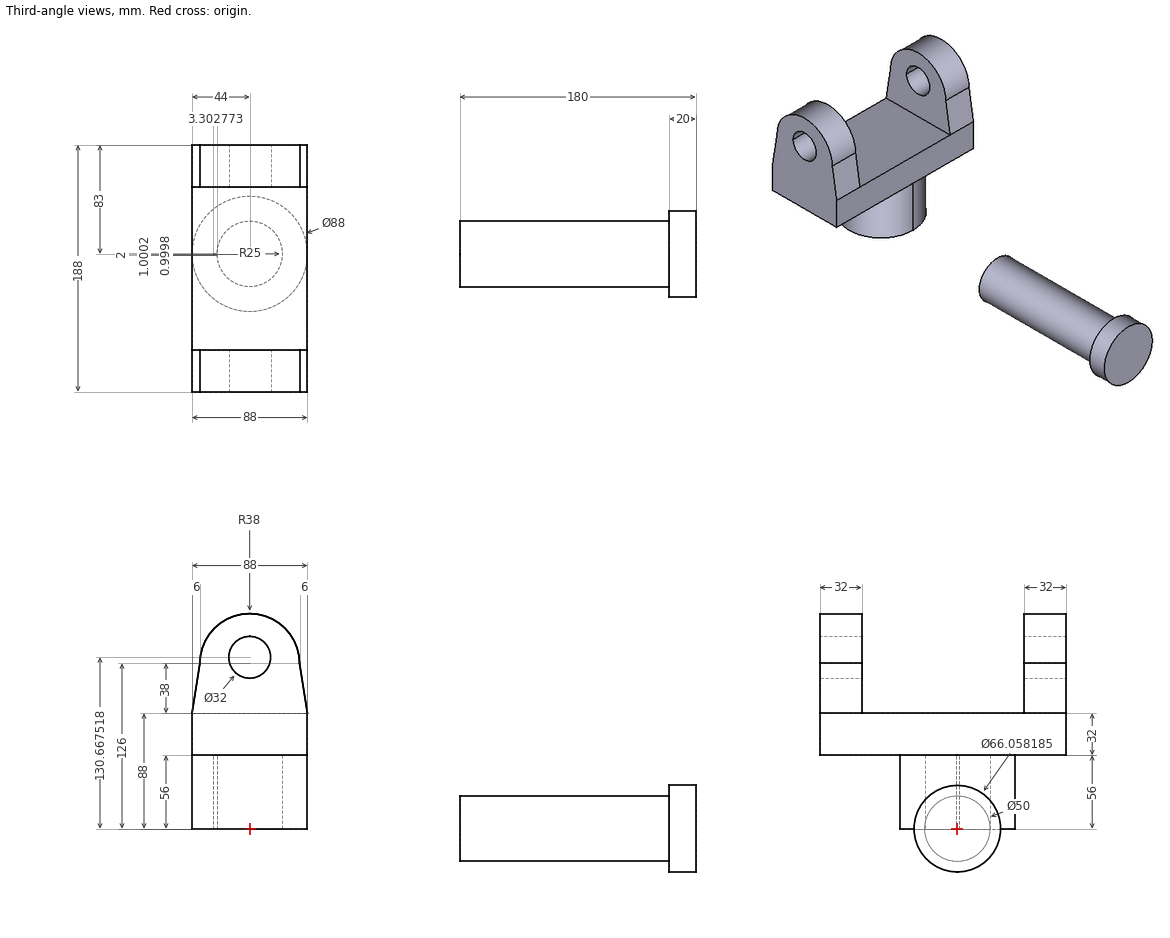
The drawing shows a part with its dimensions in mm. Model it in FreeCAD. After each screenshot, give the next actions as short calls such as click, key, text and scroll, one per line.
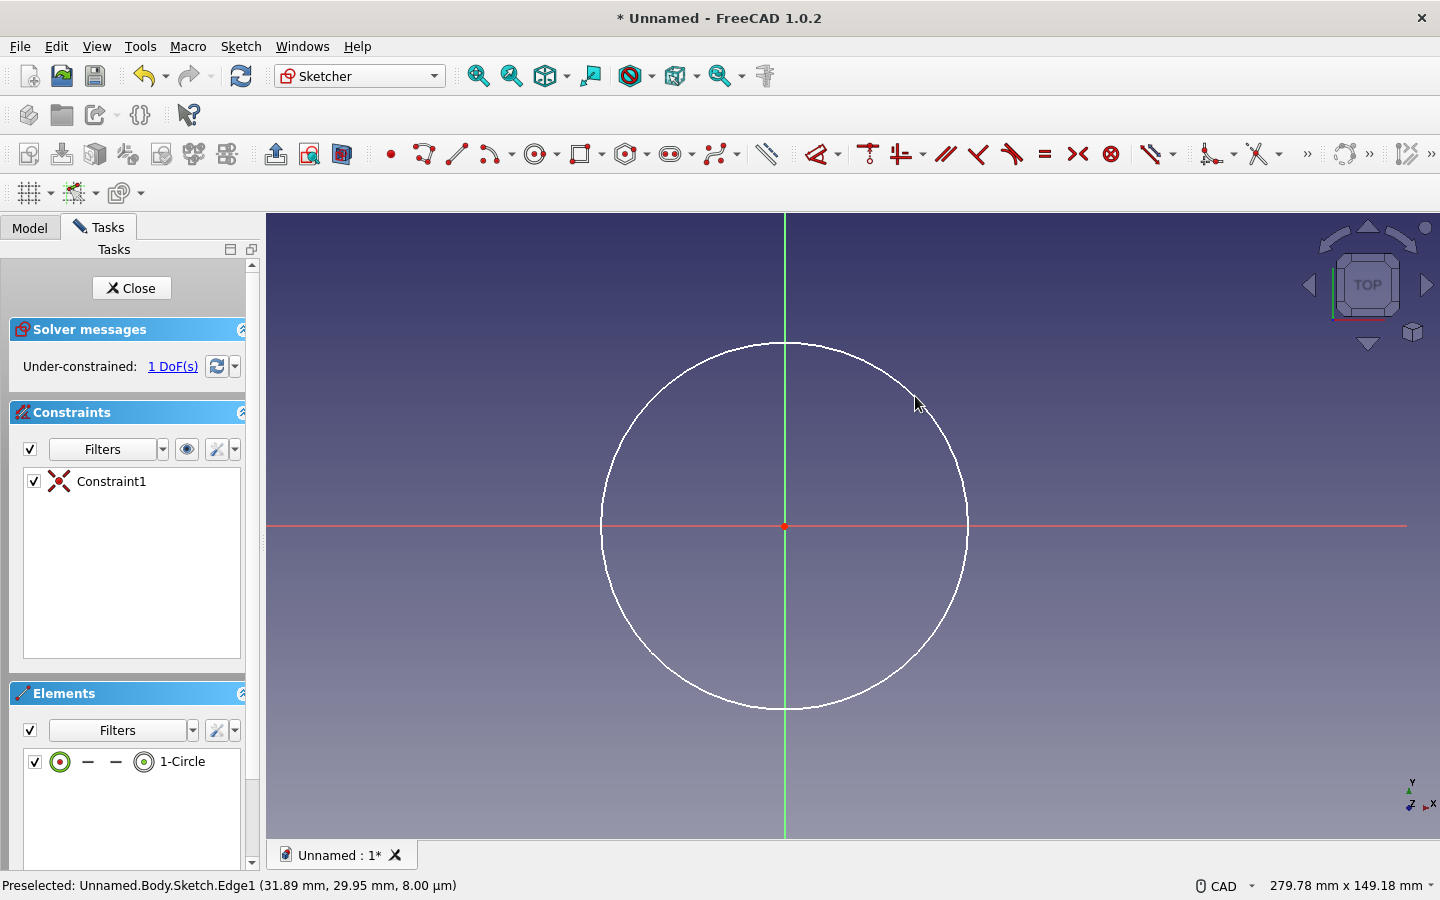
click(816, 154)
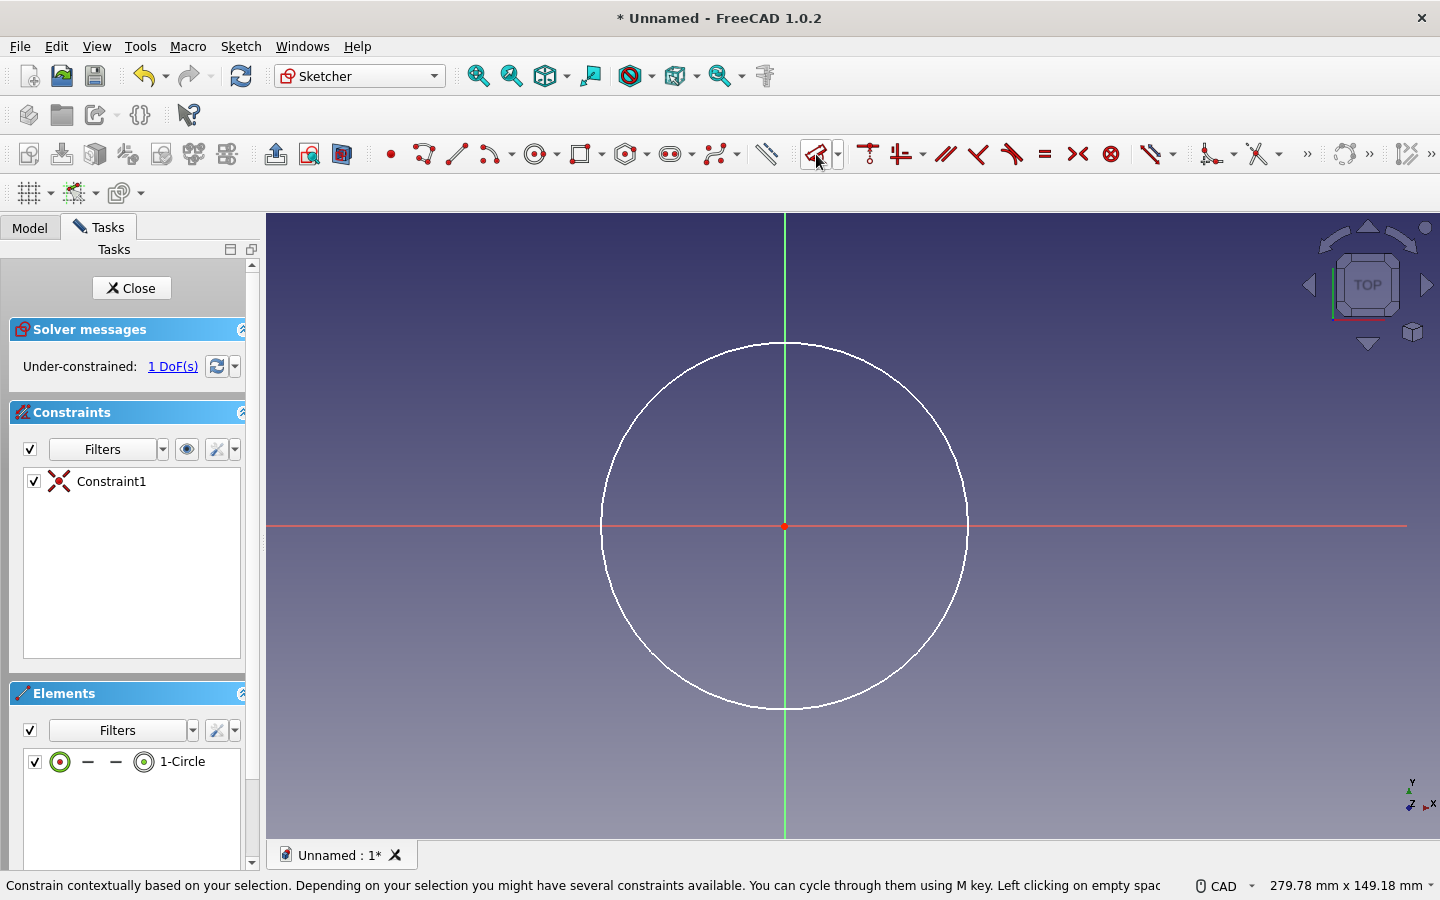
click(914, 396)
click(937, 373)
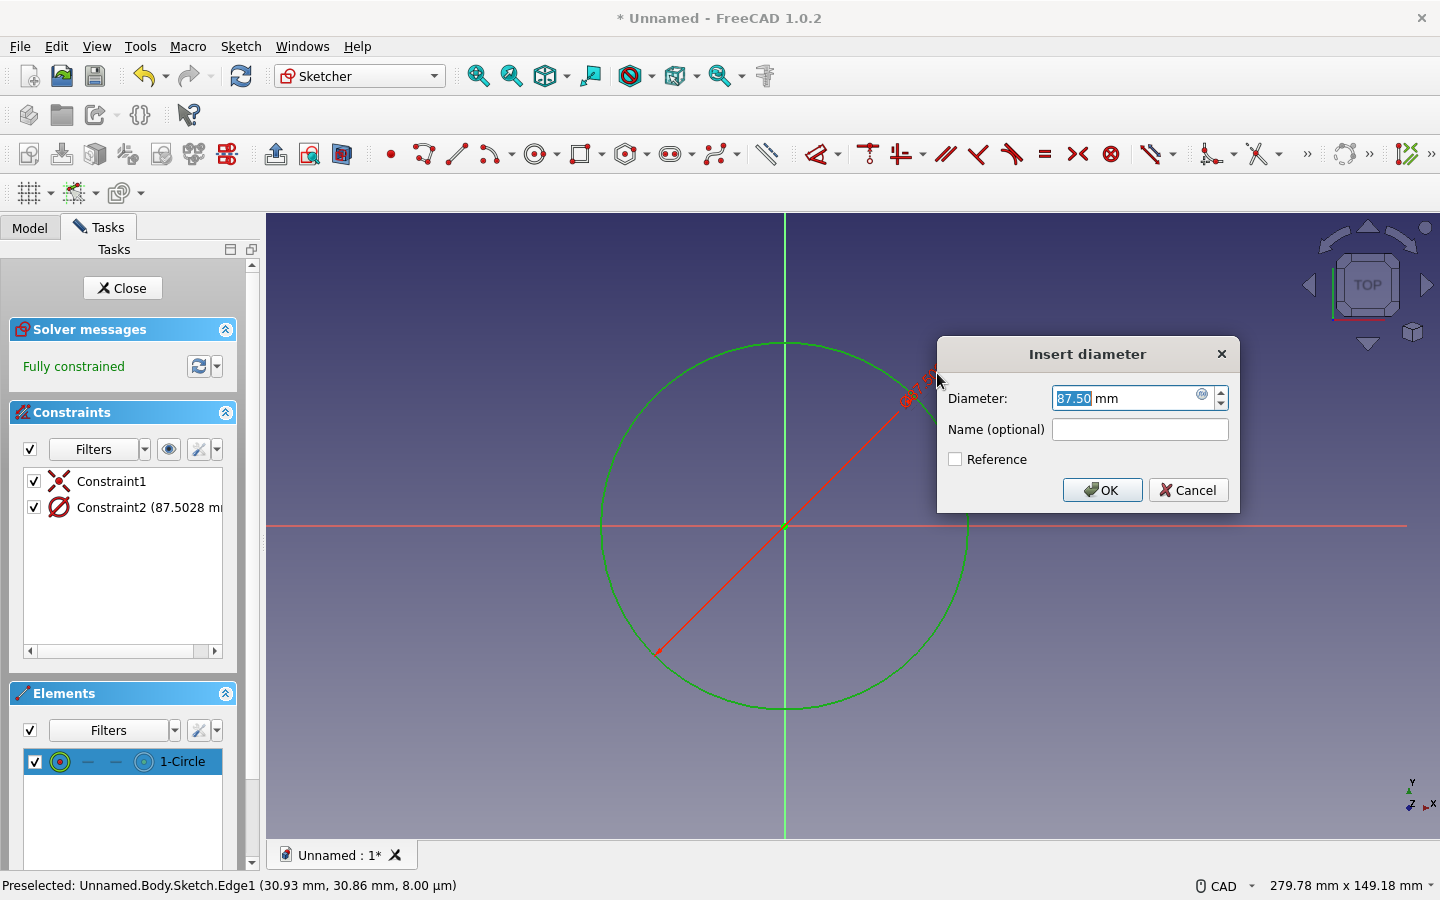
text(88)
key(Return)
key(Escape)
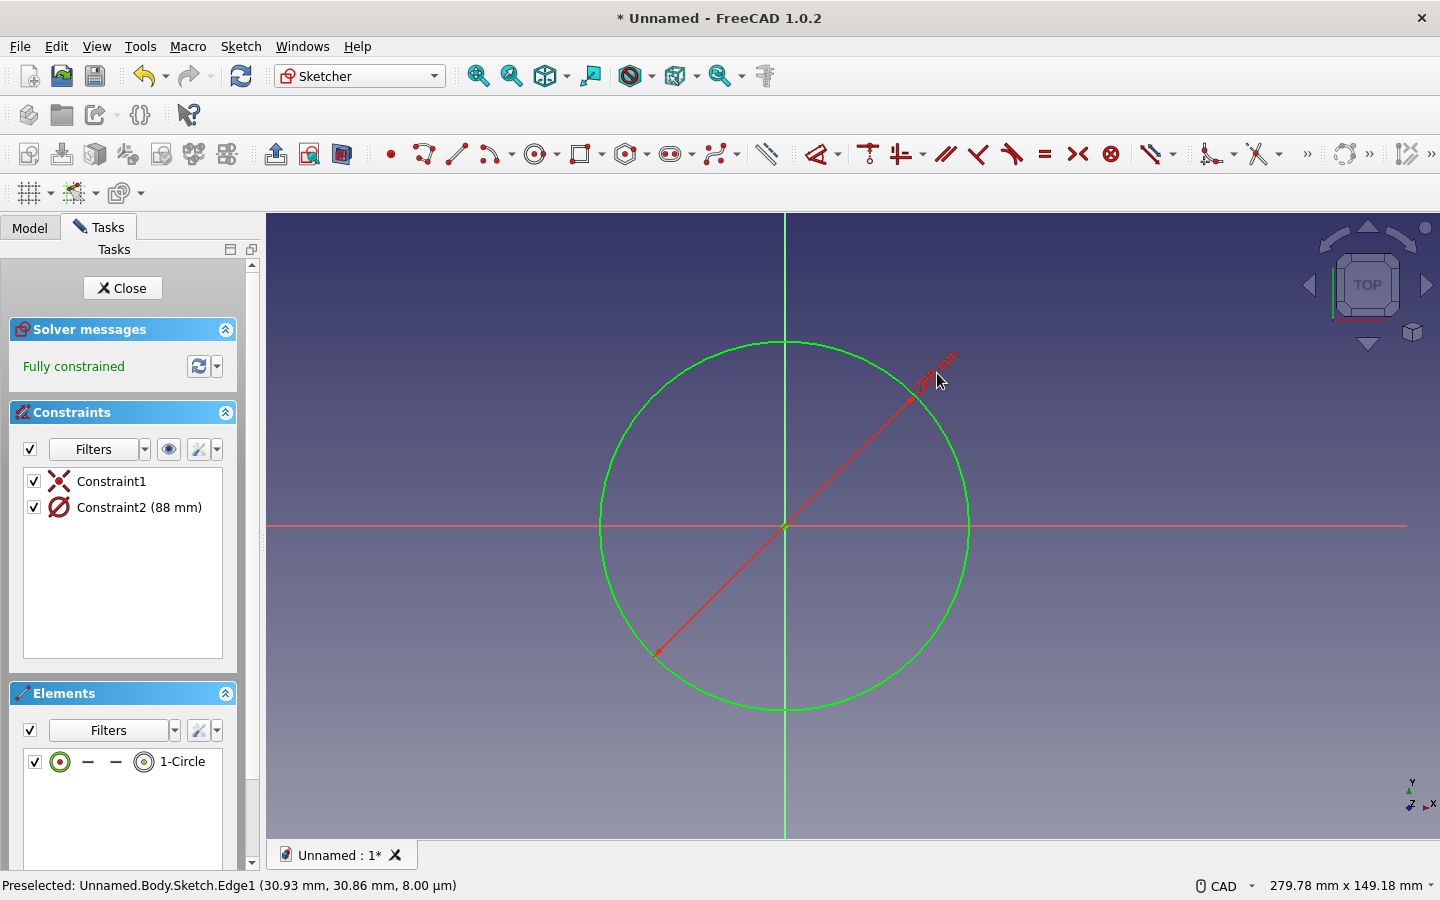
click(123, 288)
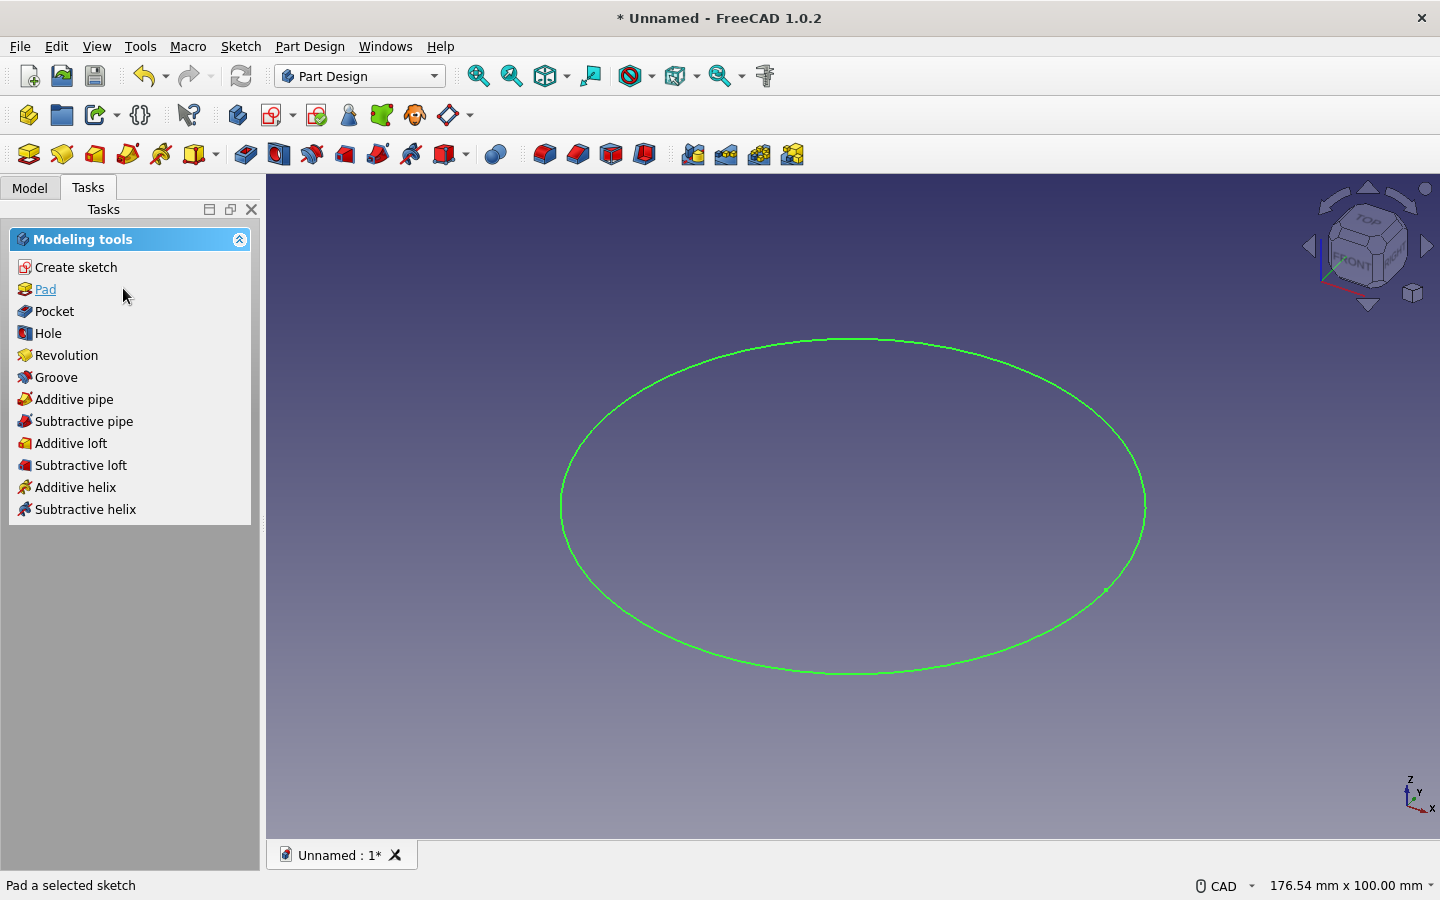
click(29, 154)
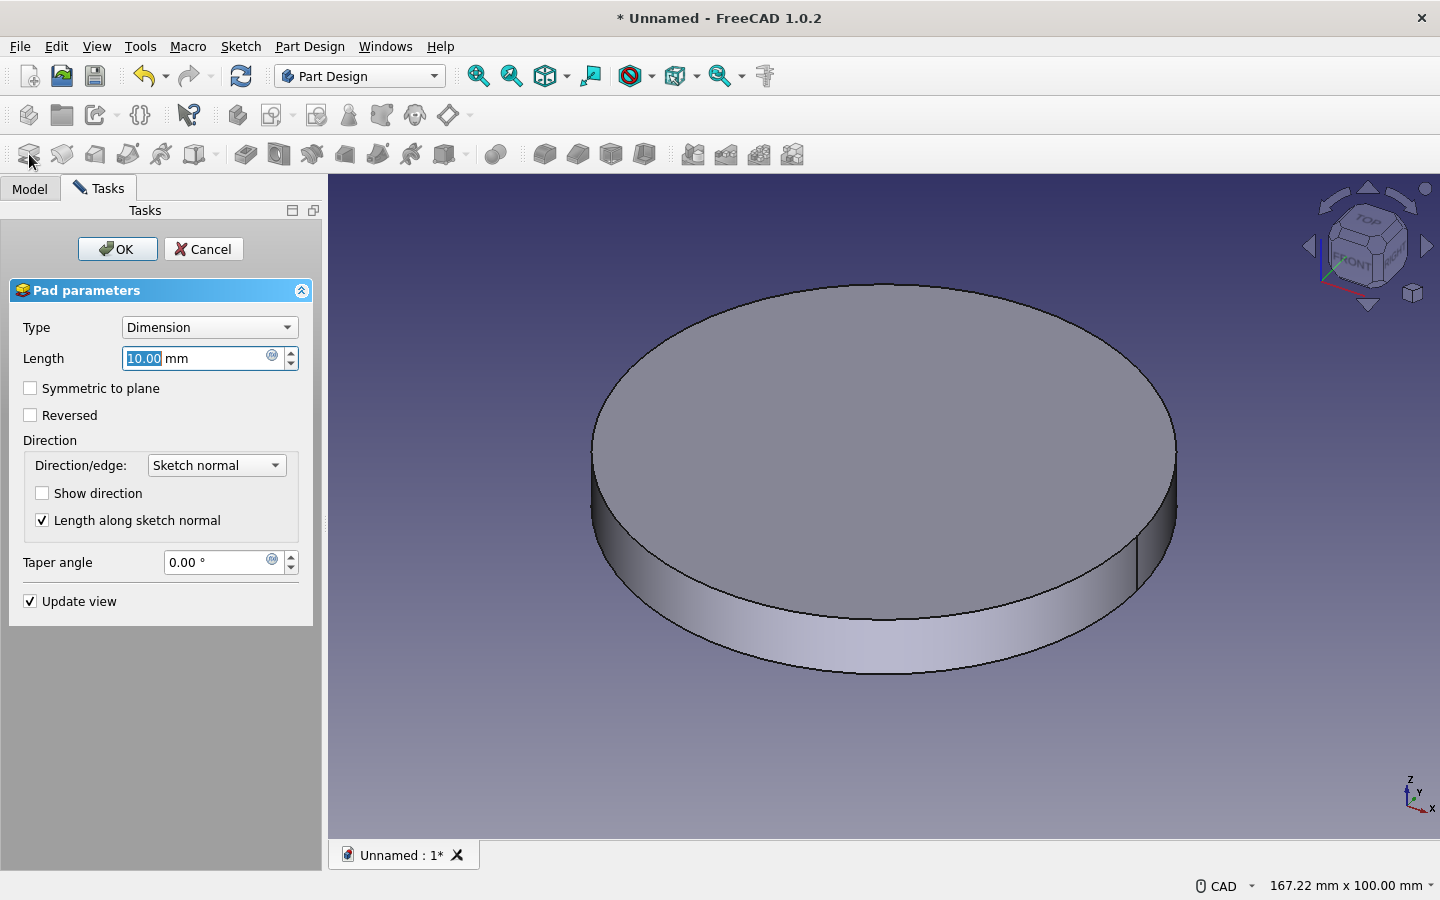
text(56)
key(Tab)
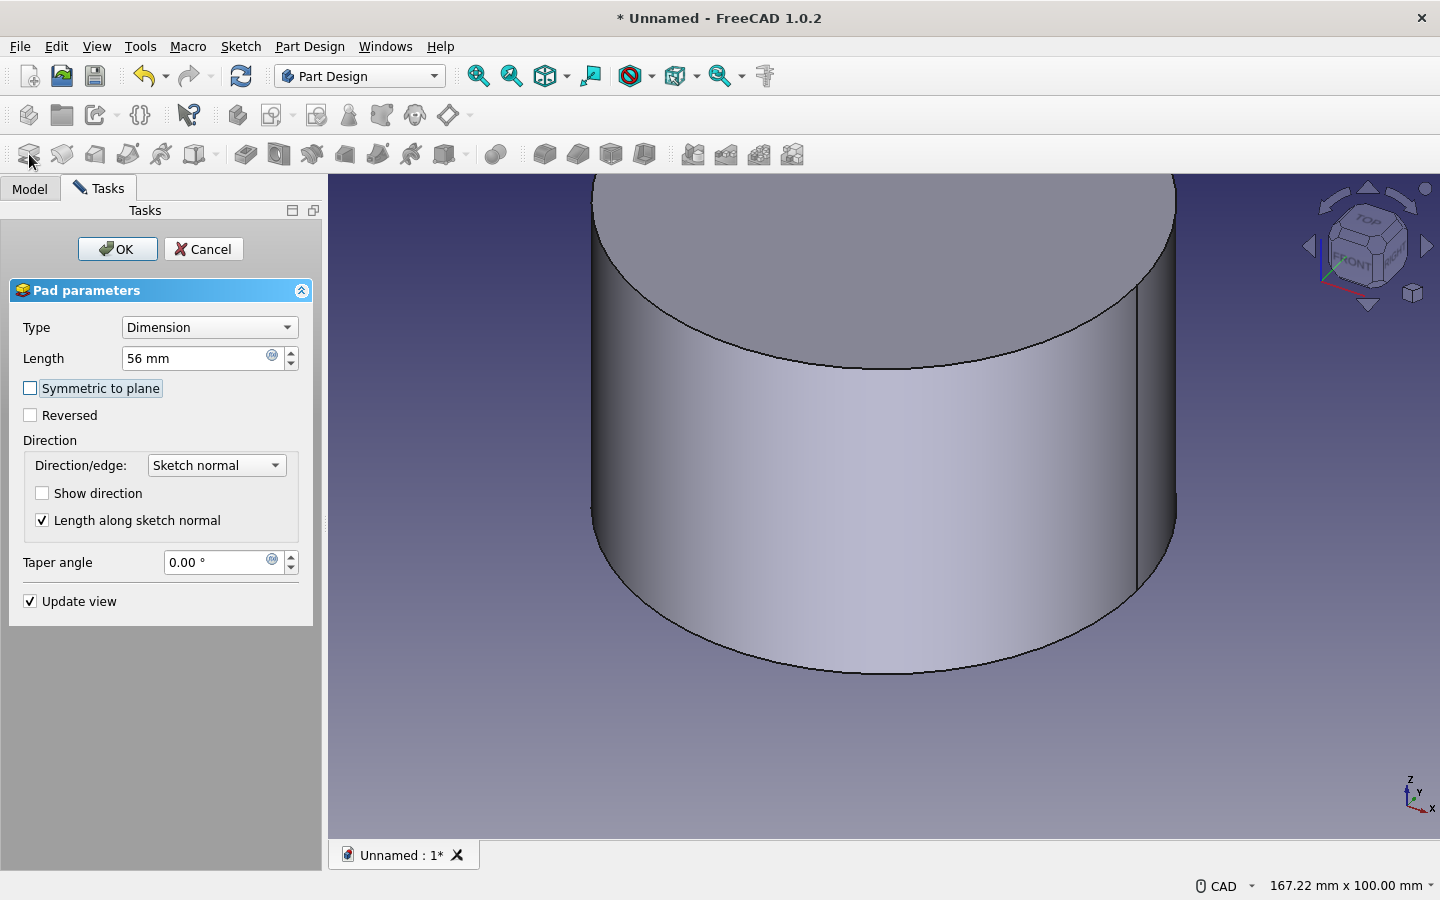
click(118, 249)